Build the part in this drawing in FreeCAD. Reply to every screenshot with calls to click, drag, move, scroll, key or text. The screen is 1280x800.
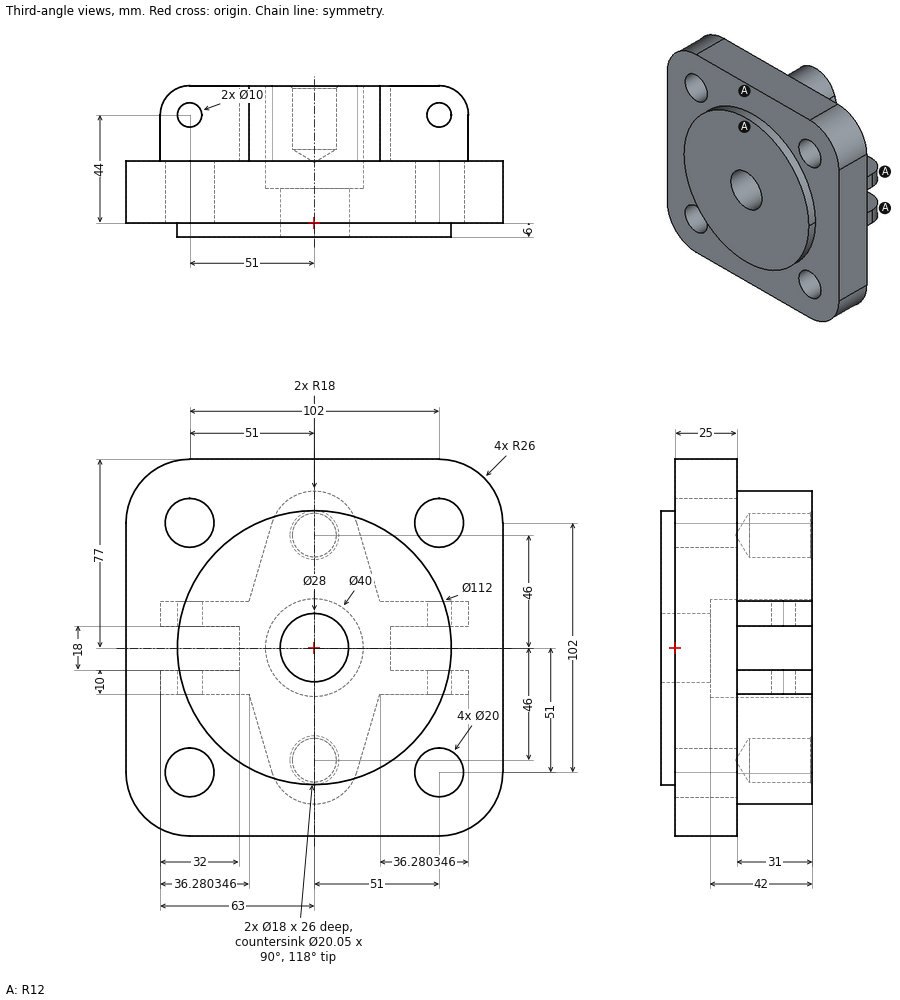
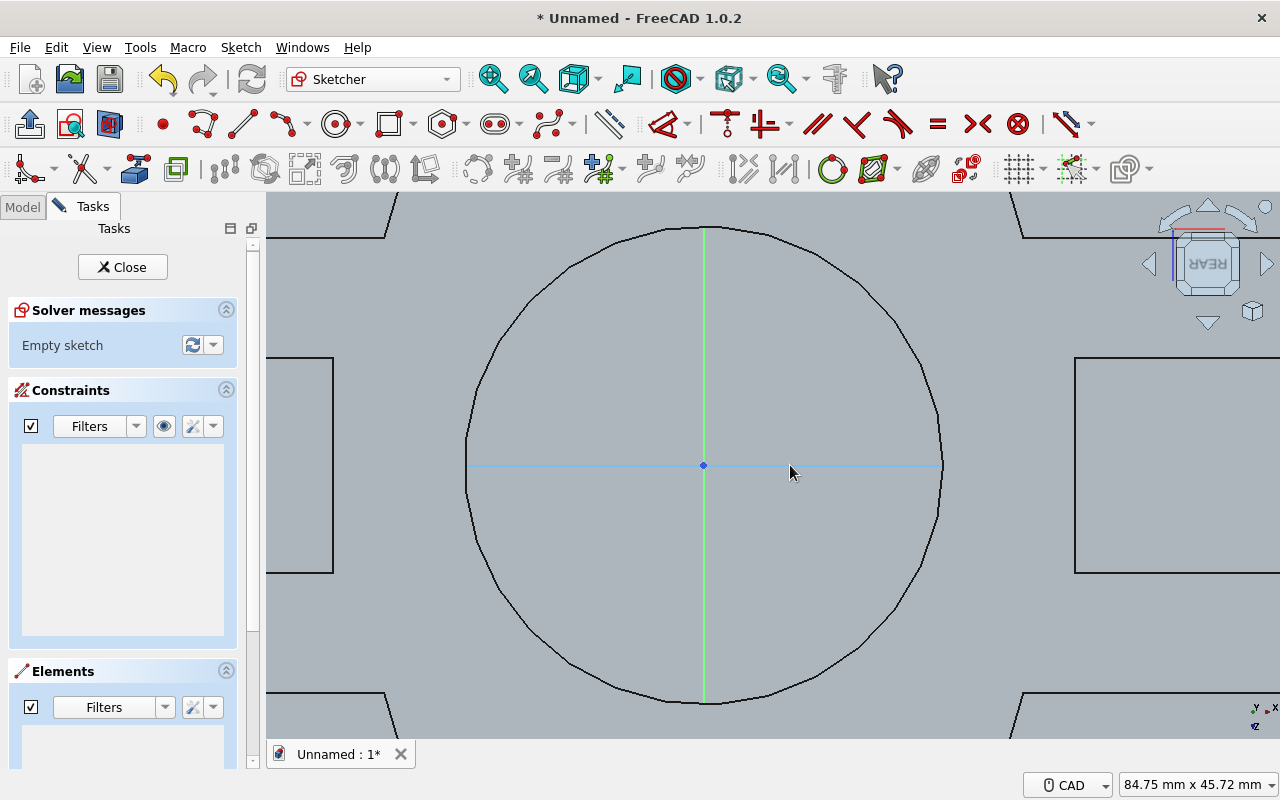
key(g)
key(c)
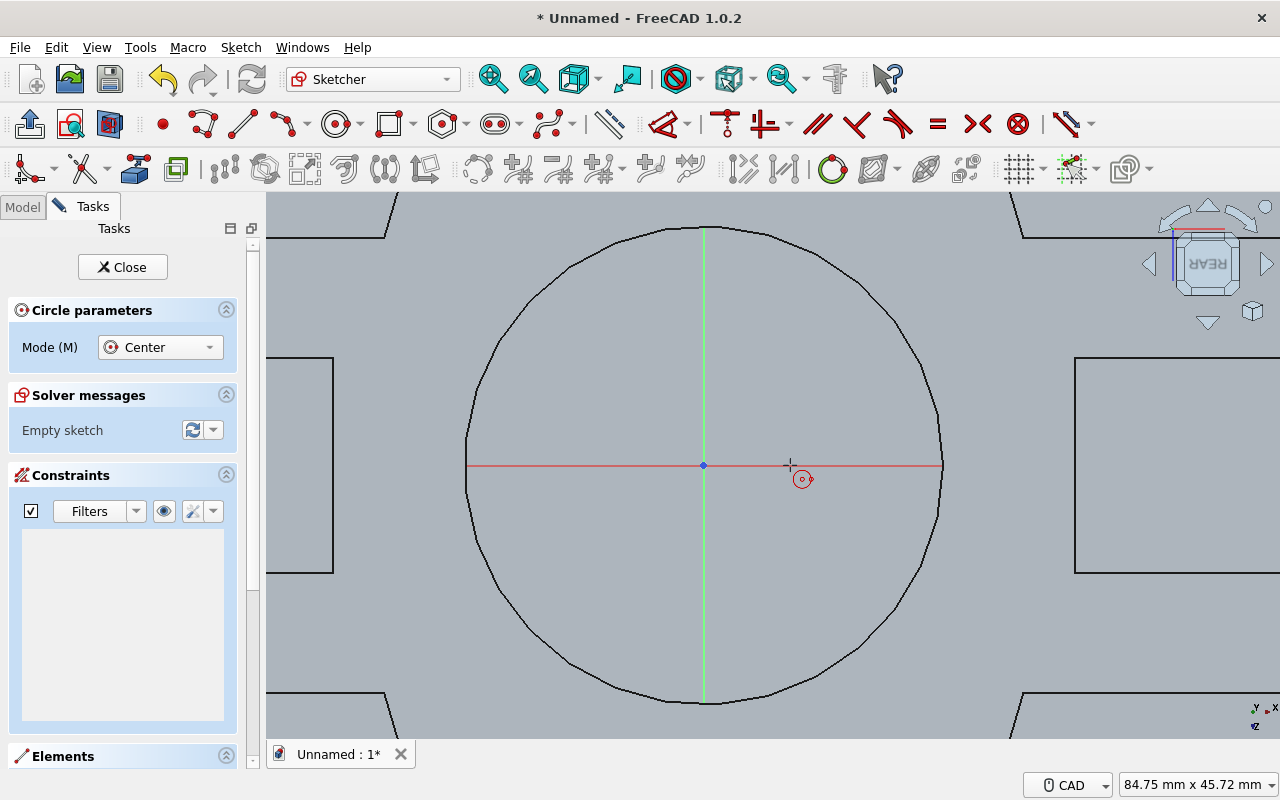
click(704, 465)
click(822, 347)
key(Escape)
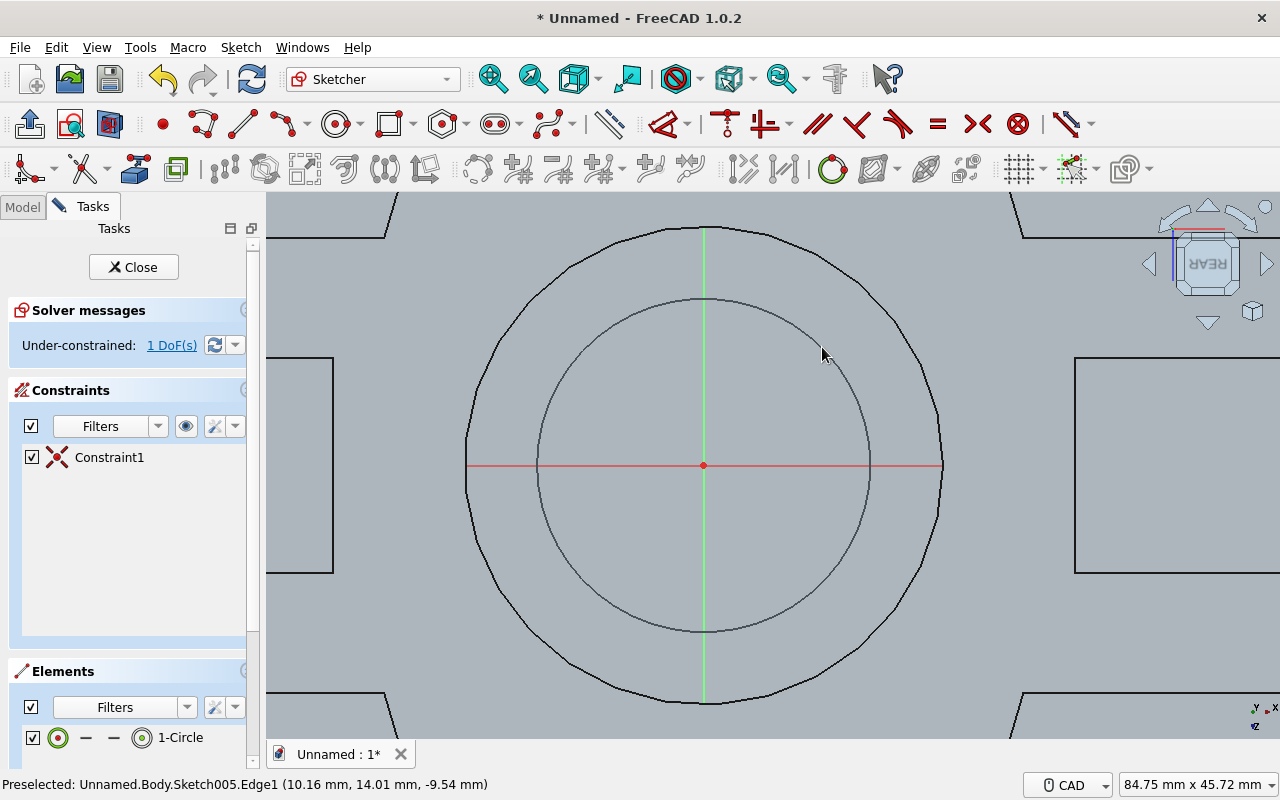
key(d)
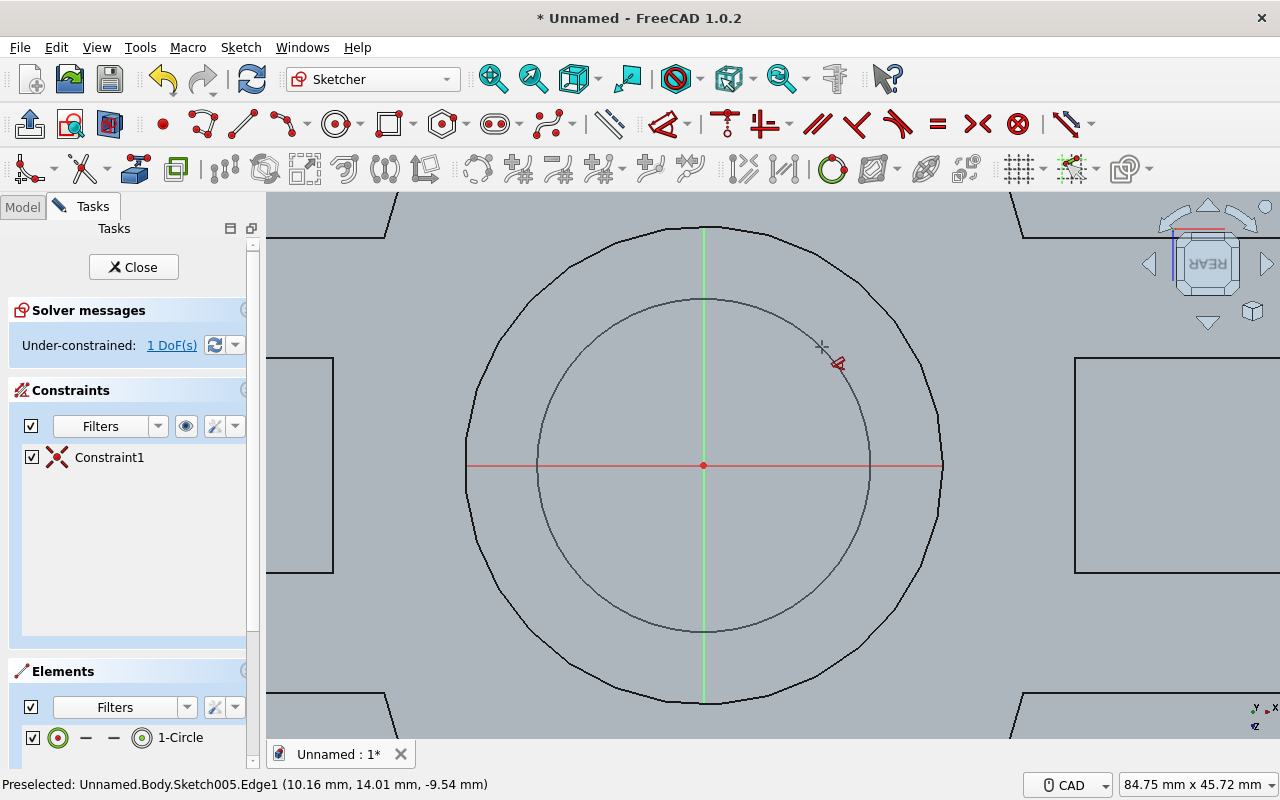
click(821, 347)
click(844, 324)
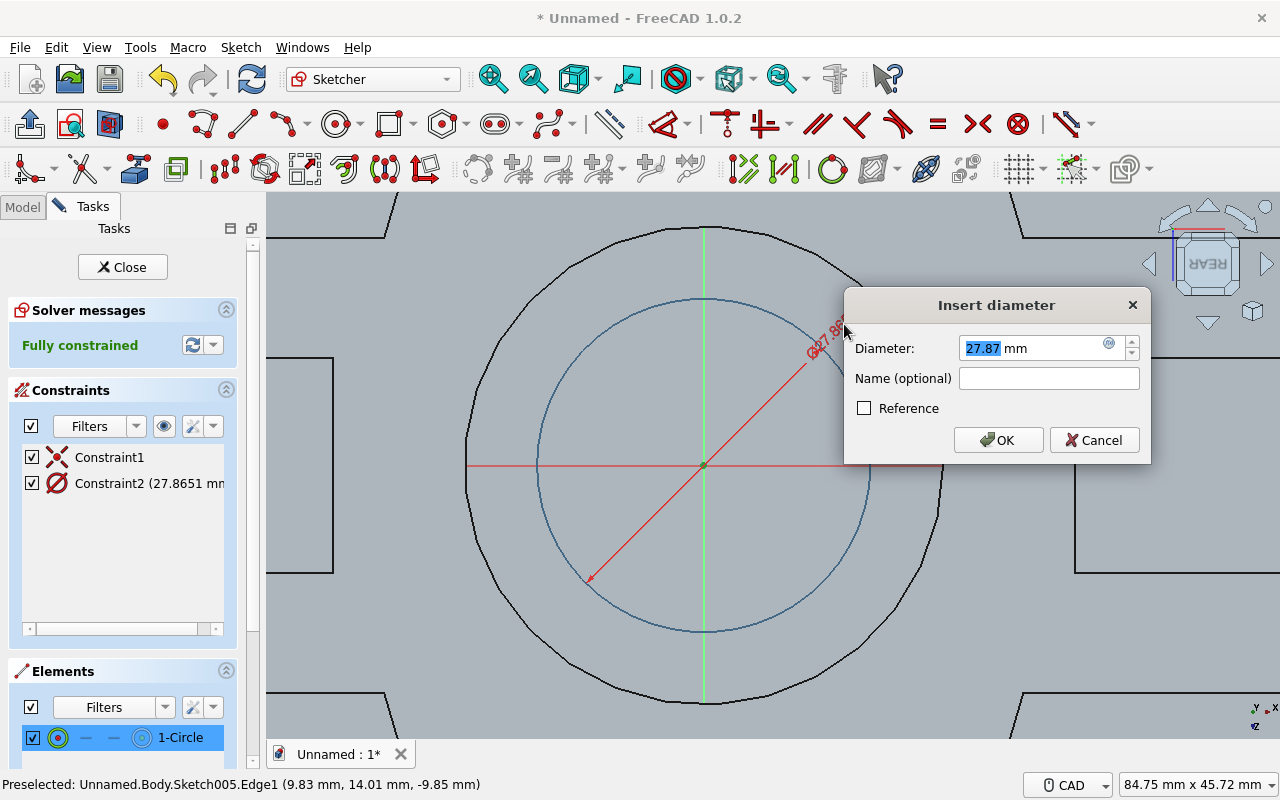
text(28)
key(Return)
key(Escape)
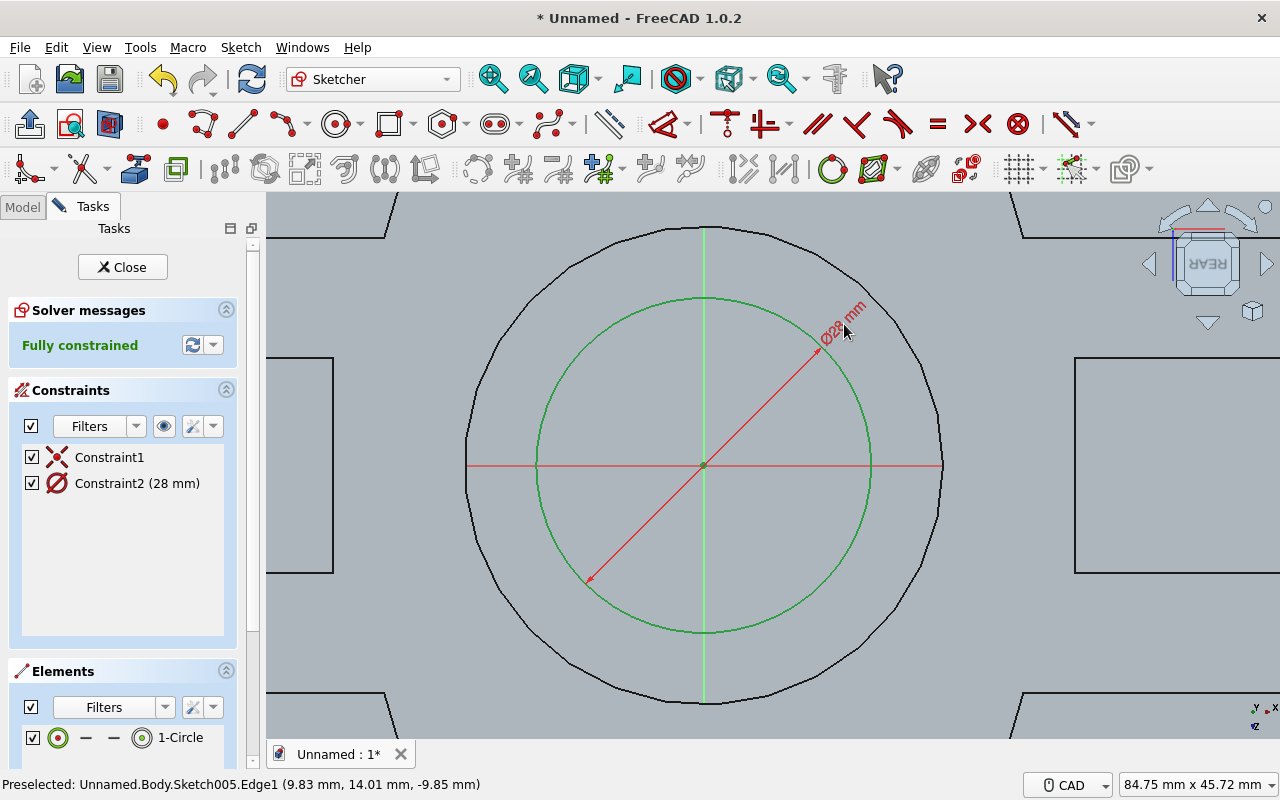
click(123, 267)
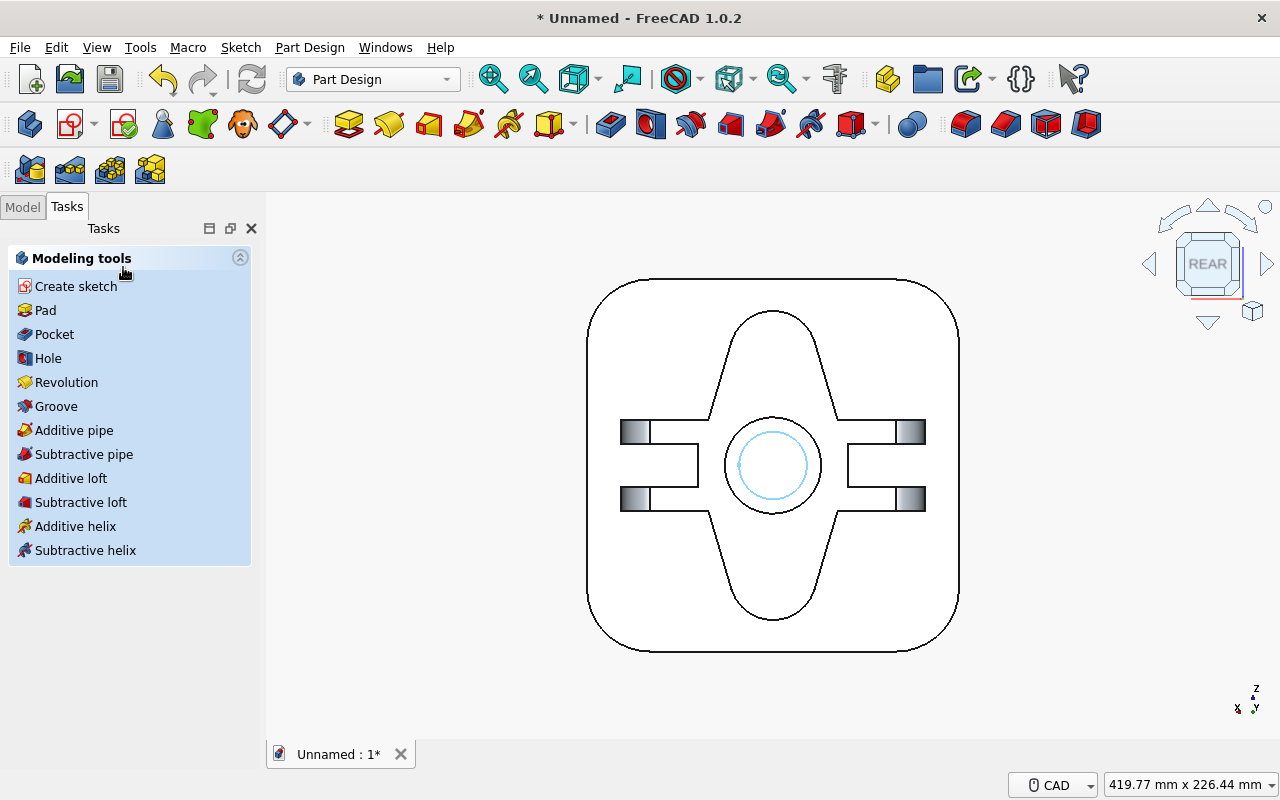
click(612, 124)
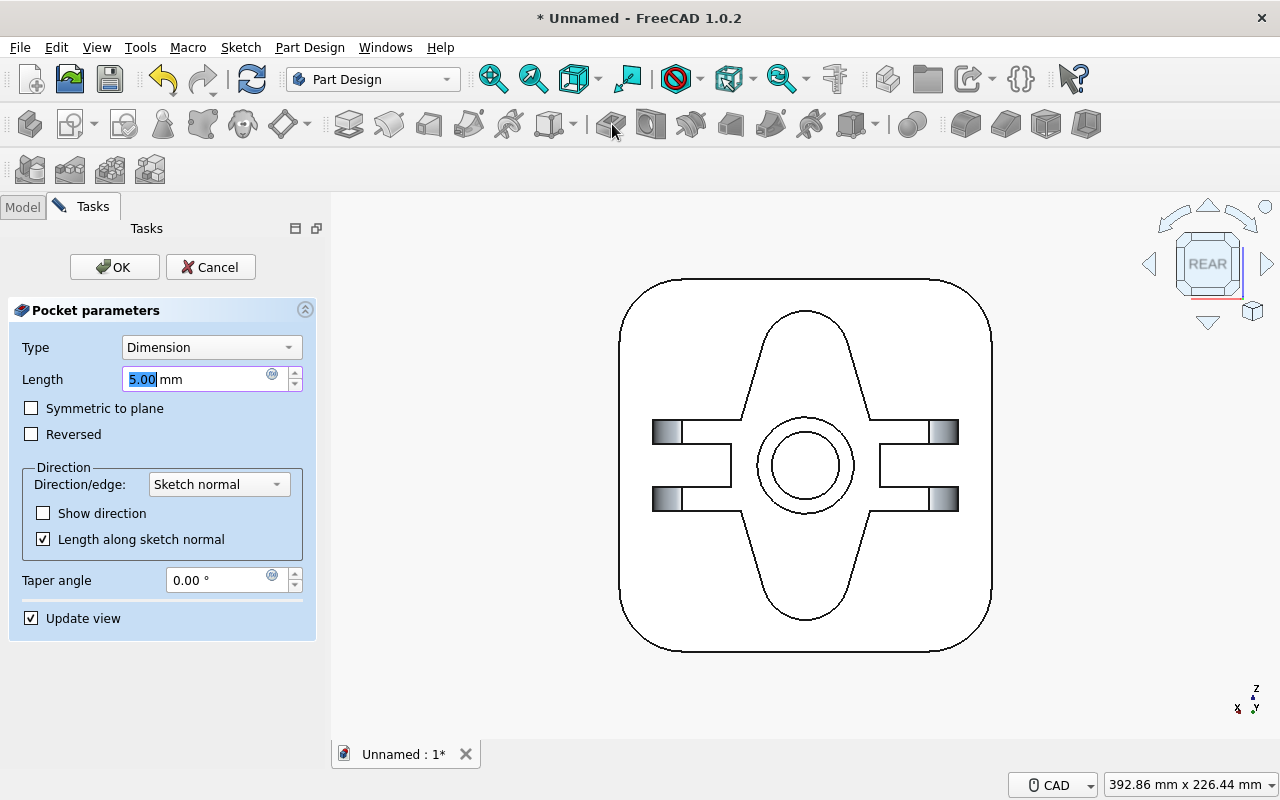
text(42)
key(Tab)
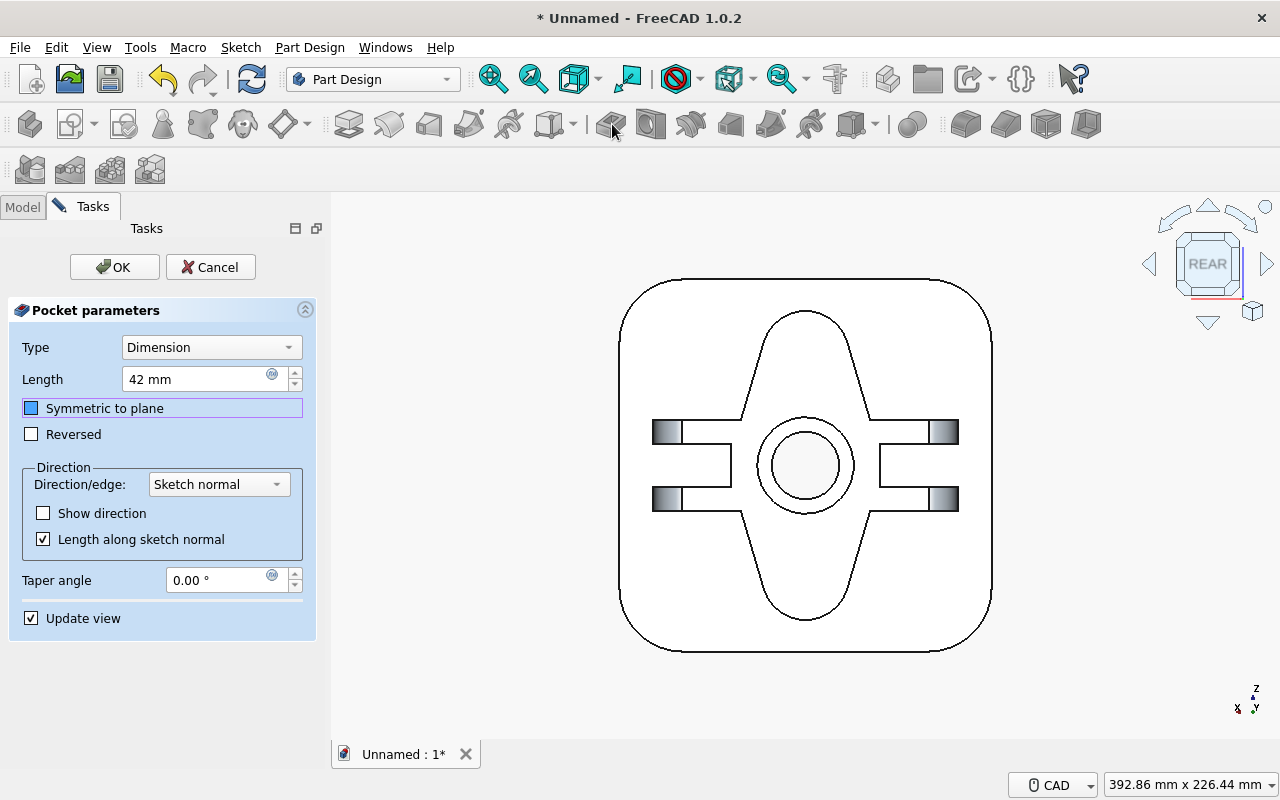
click(115, 267)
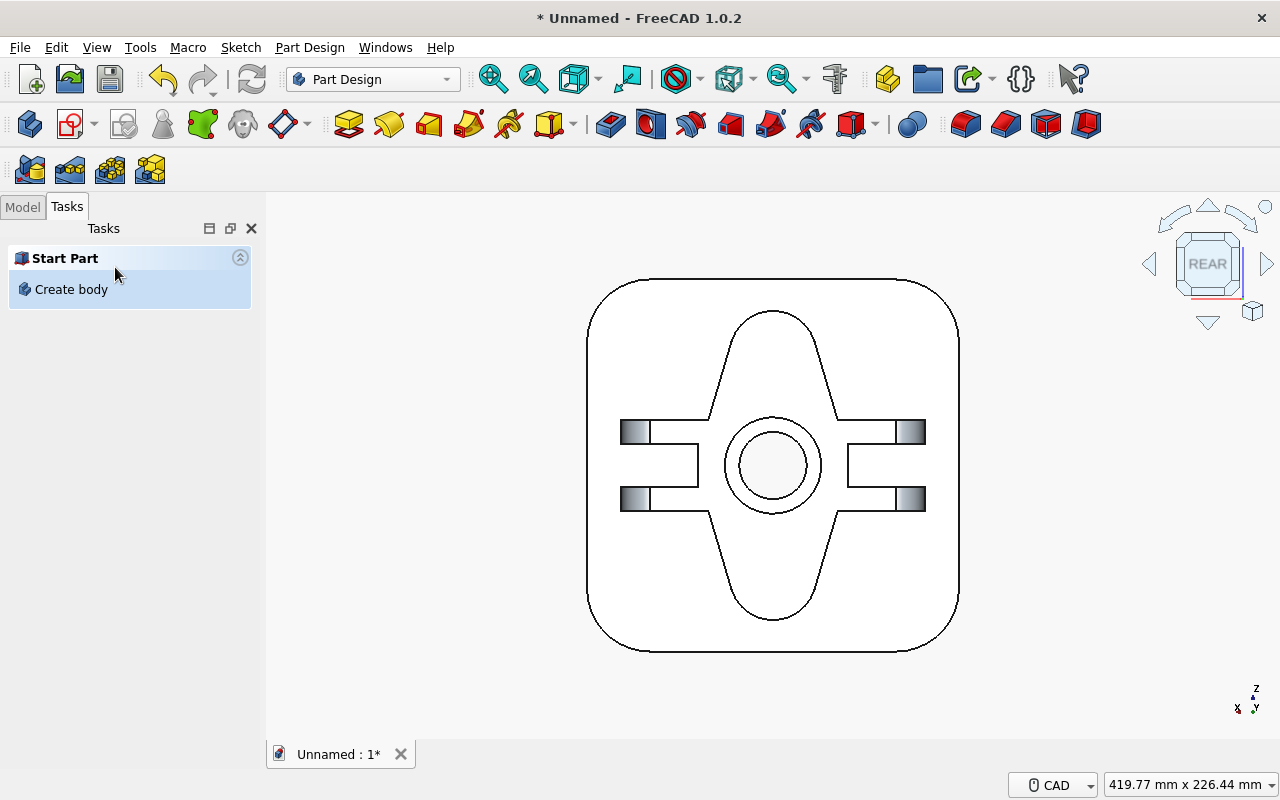
click(773, 376)